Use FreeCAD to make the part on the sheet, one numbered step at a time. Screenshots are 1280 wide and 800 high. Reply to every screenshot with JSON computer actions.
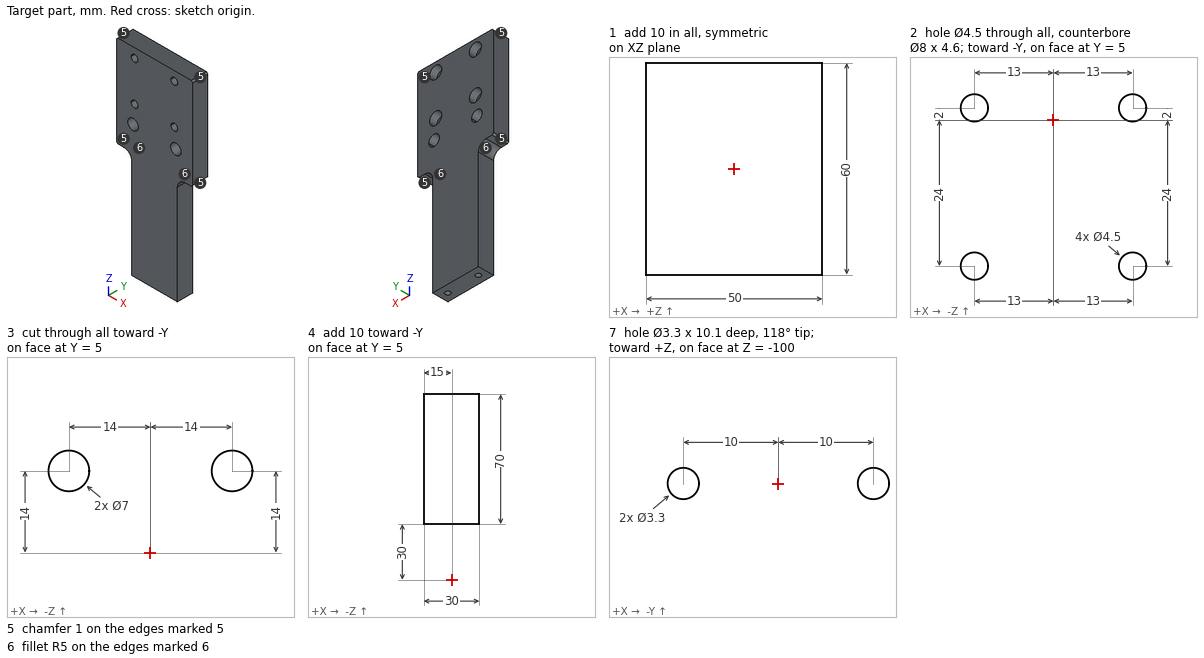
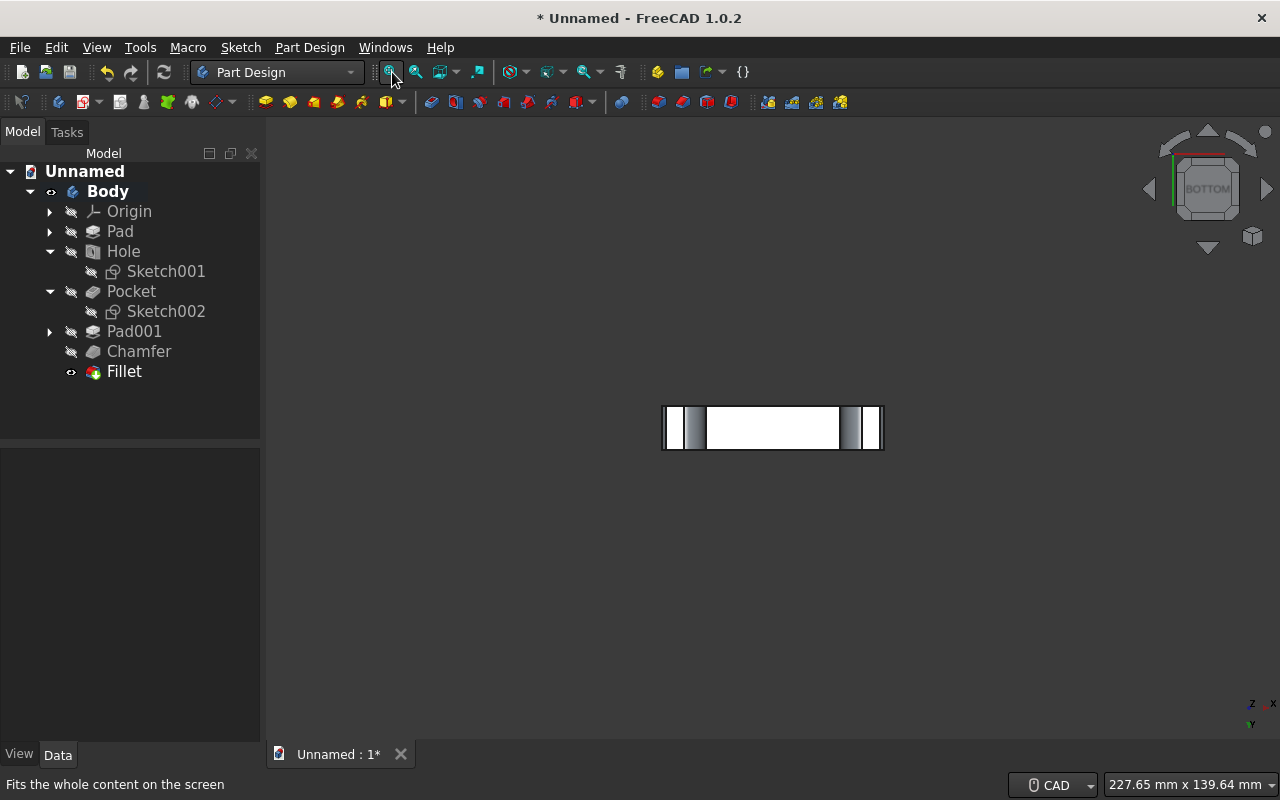
{"action": "left_click", "coordinate": [811, 427]}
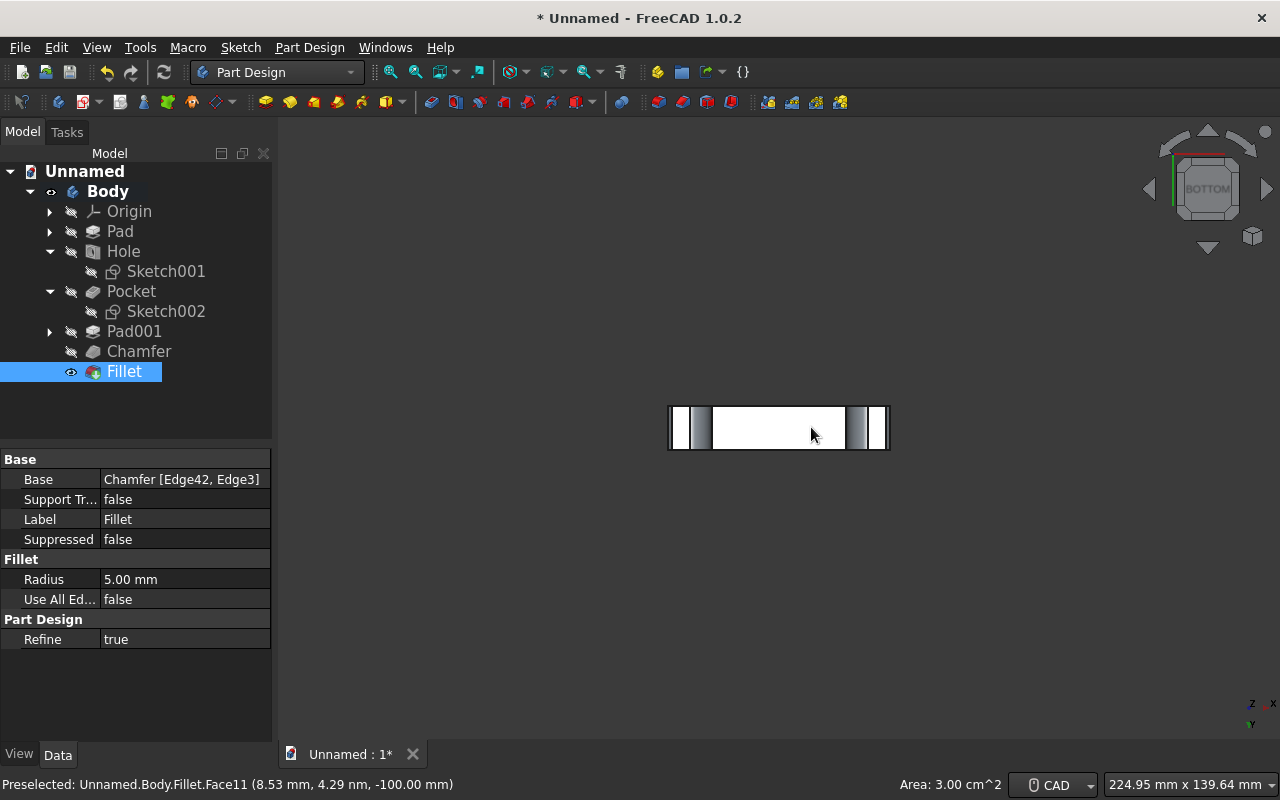
{"action": "left_click", "coordinate": [84, 102]}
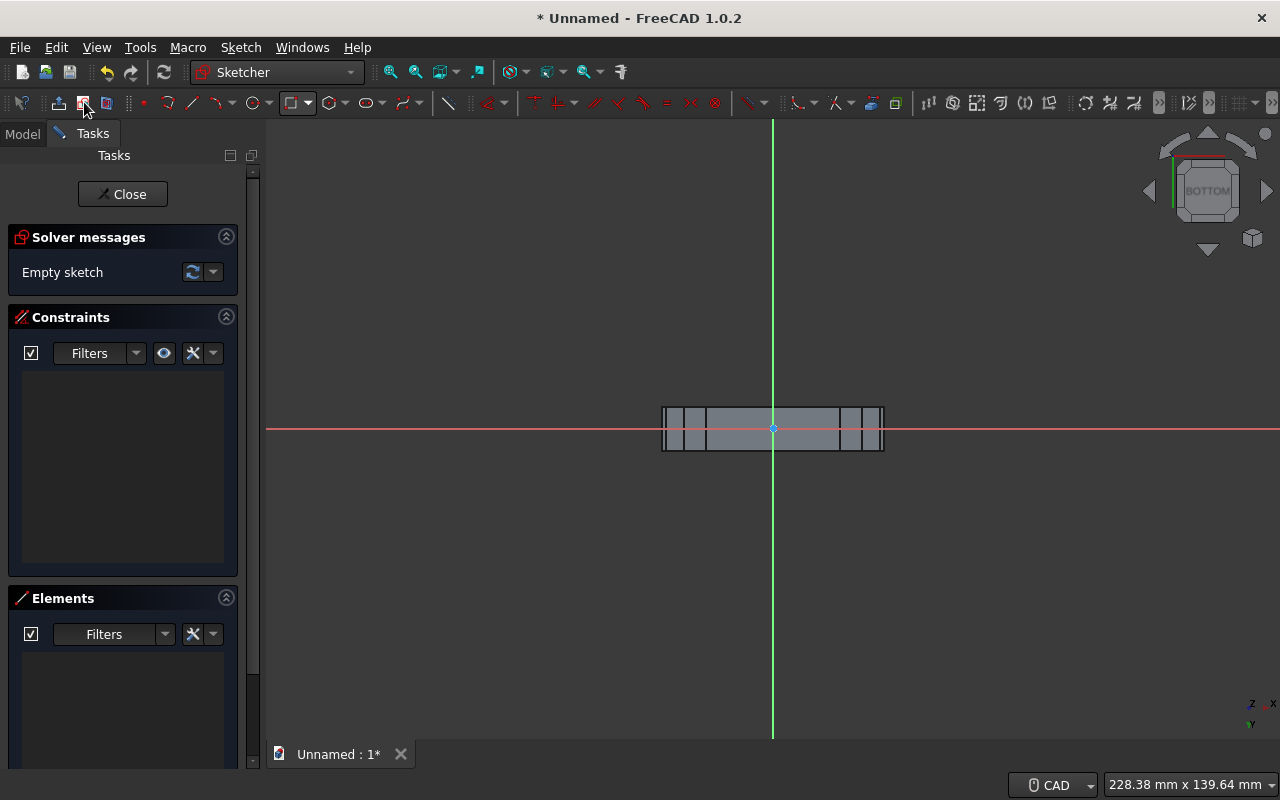
{"action": "scroll", "coordinate": [787, 429], "scroll_direction": "up", "scroll_amount": 9}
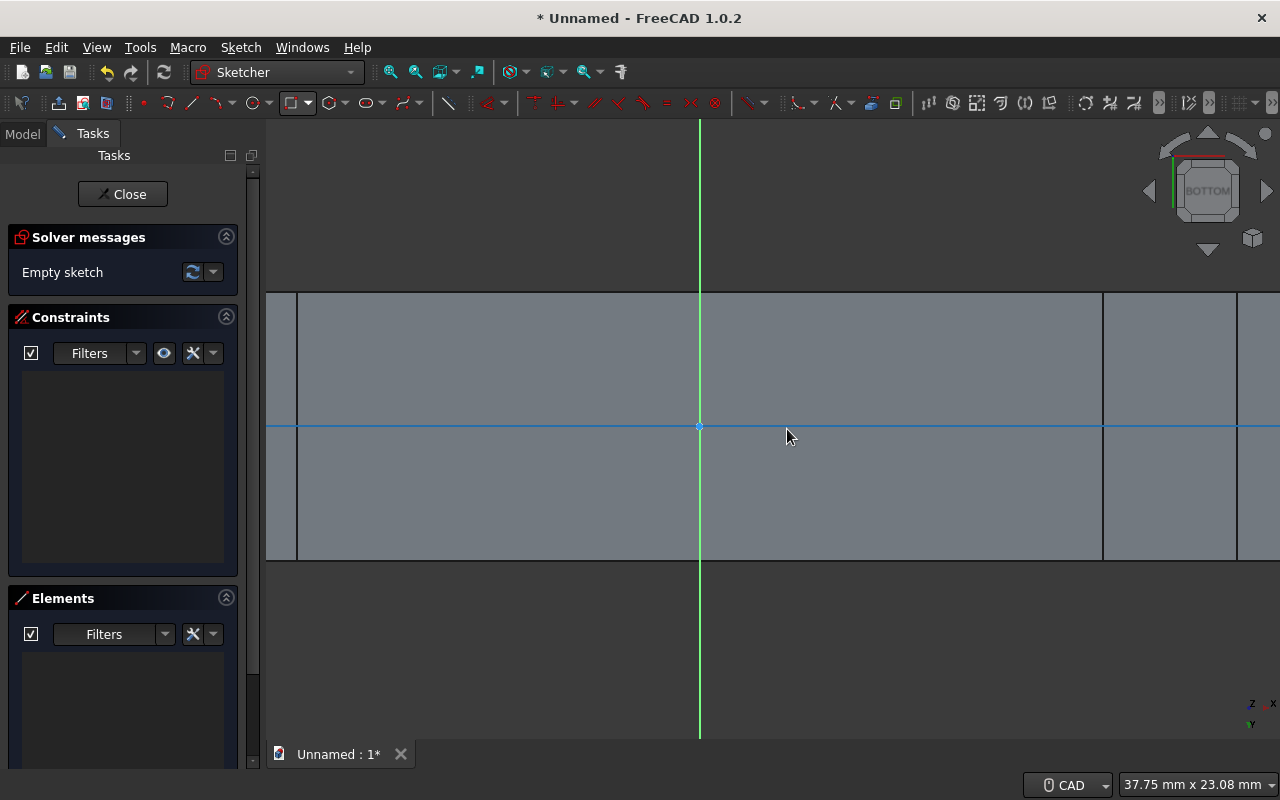
{"action": "left_click", "coordinate": [254, 104]}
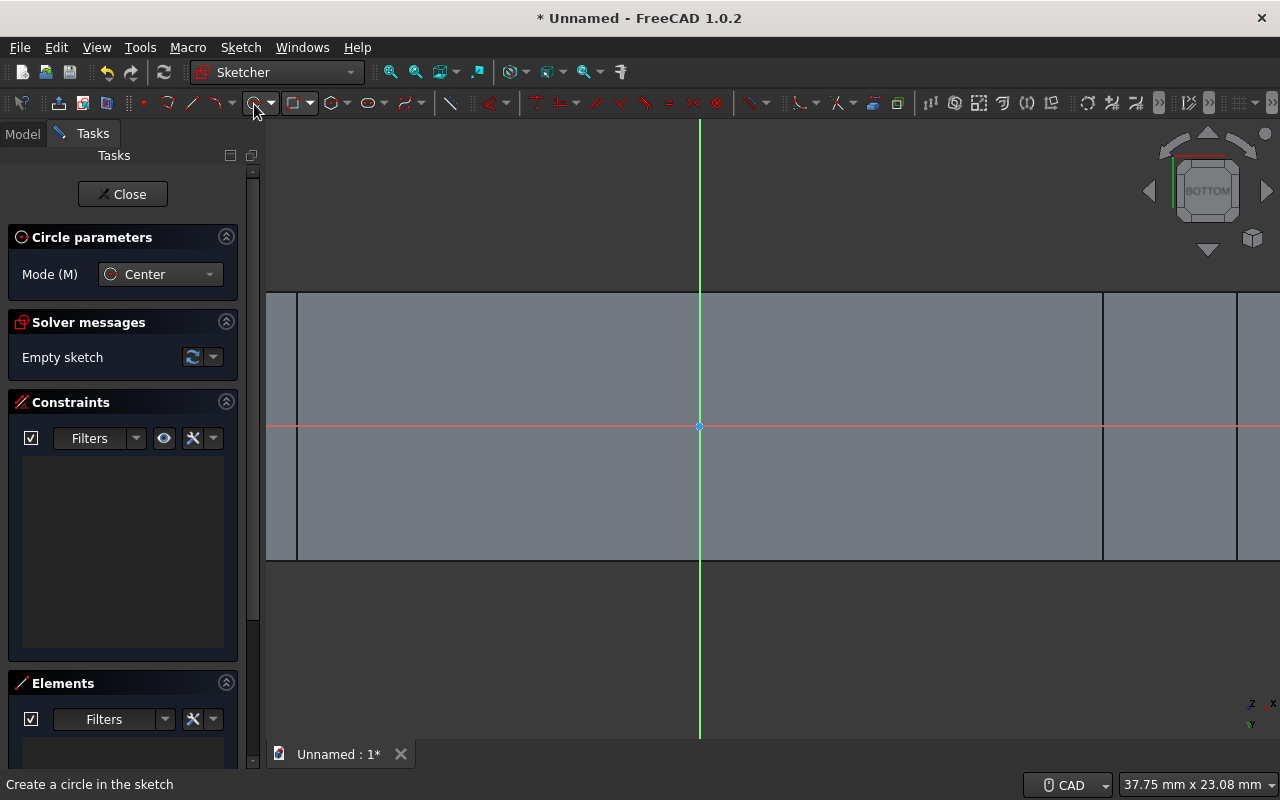
{"action": "left_click", "coordinate": [431, 426]}
{"action": "mouse_move", "coordinate": [462, 395]}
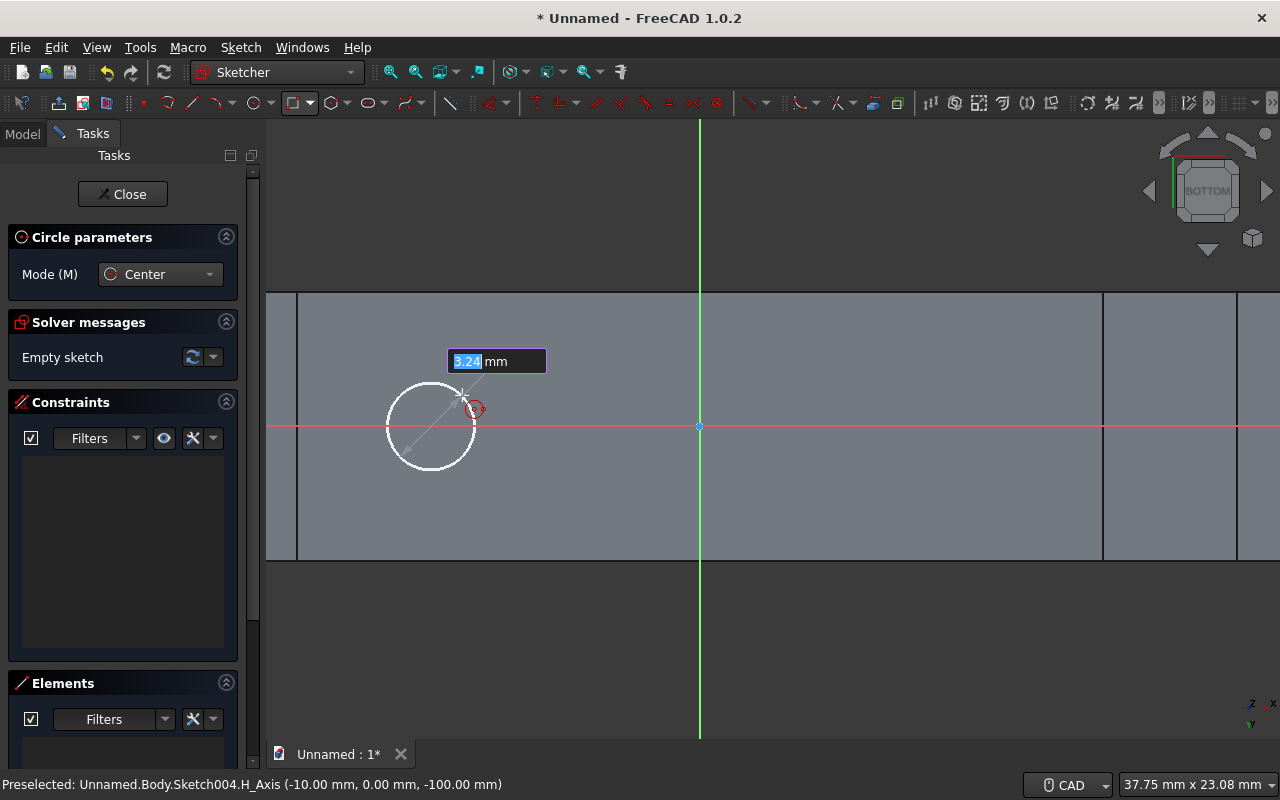
{"action": "type", "text": "3.3"}
{"action": "key", "text": "Return"}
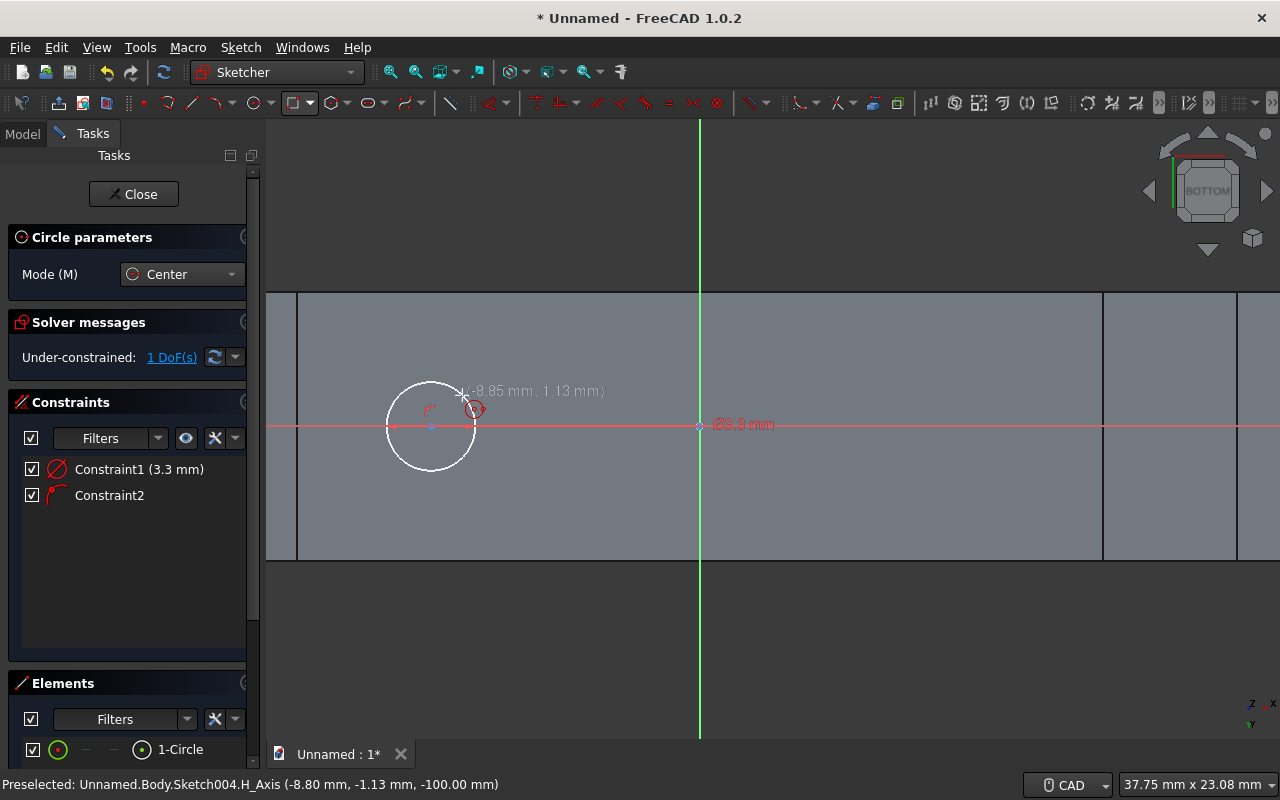
{"action": "left_click", "coordinate": [968, 426]}
{"action": "mouse_move", "coordinate": [1000, 395]}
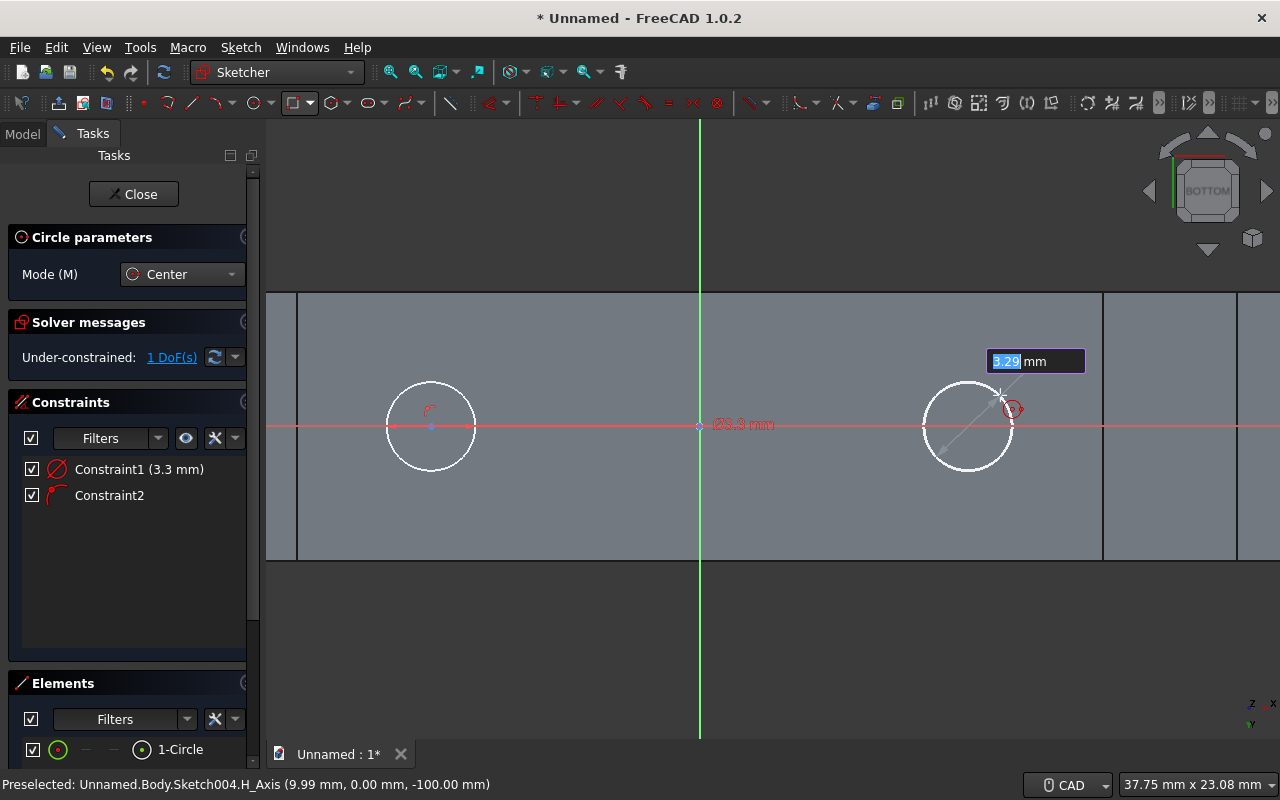
{"action": "type", "text": "3.3"}
{"action": "key", "text": "Return"}
{"action": "key", "text": "Escape"}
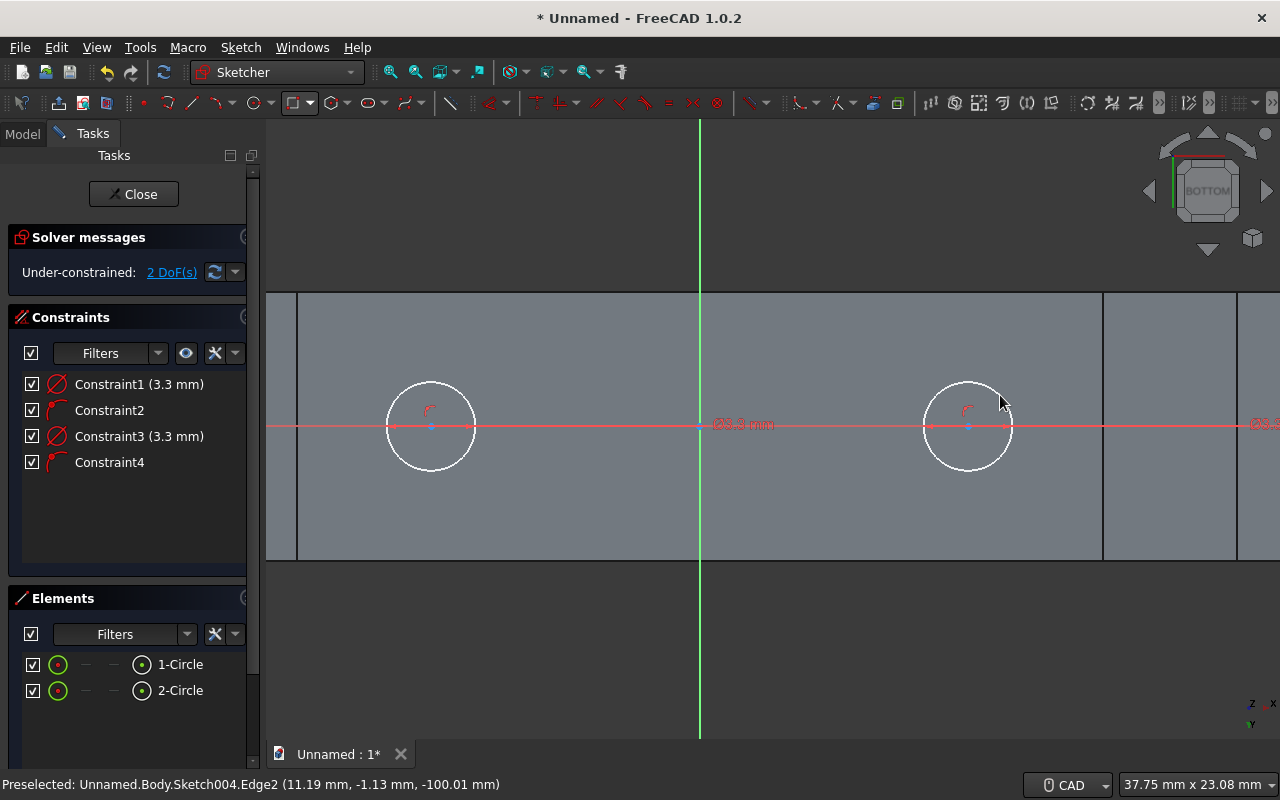
{"action": "key", "text": "d"}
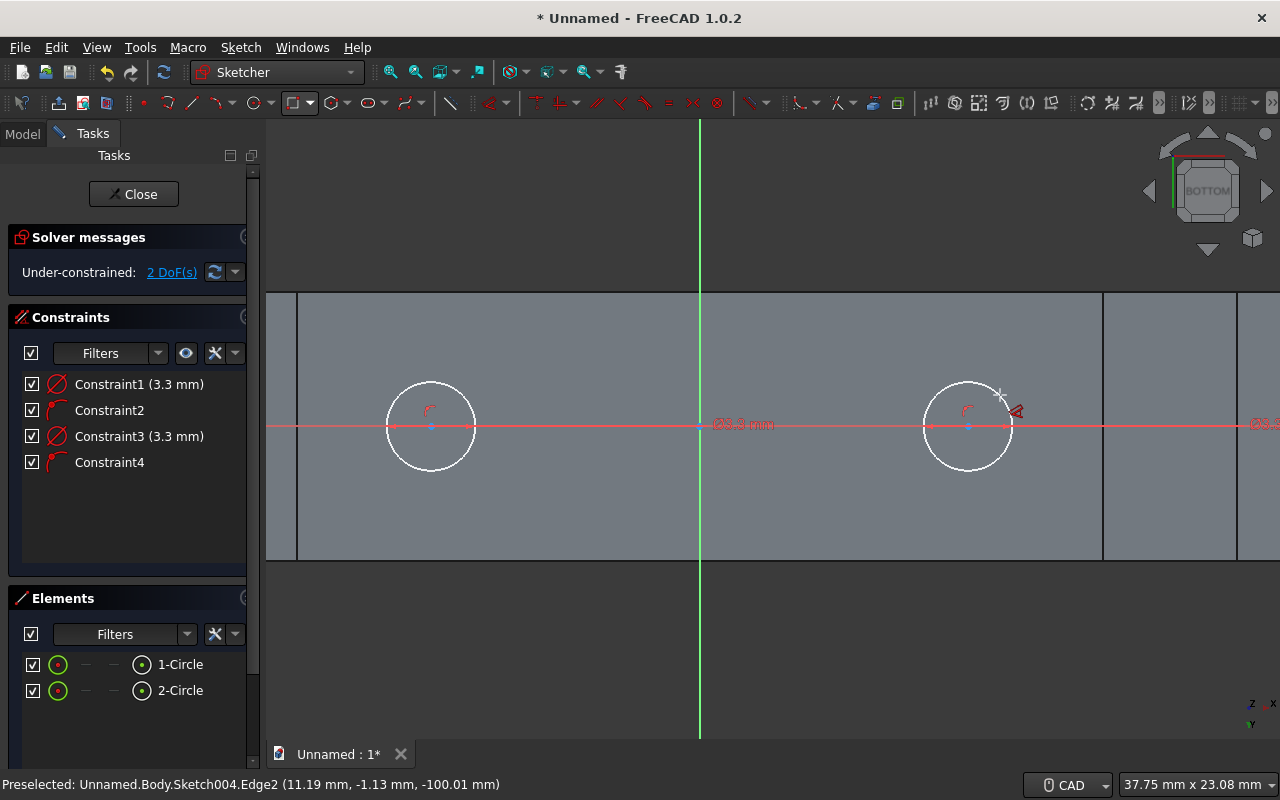
{"action": "left_click", "coordinate": [431, 426]}
{"action": "left_click", "coordinate": [565, 460]}